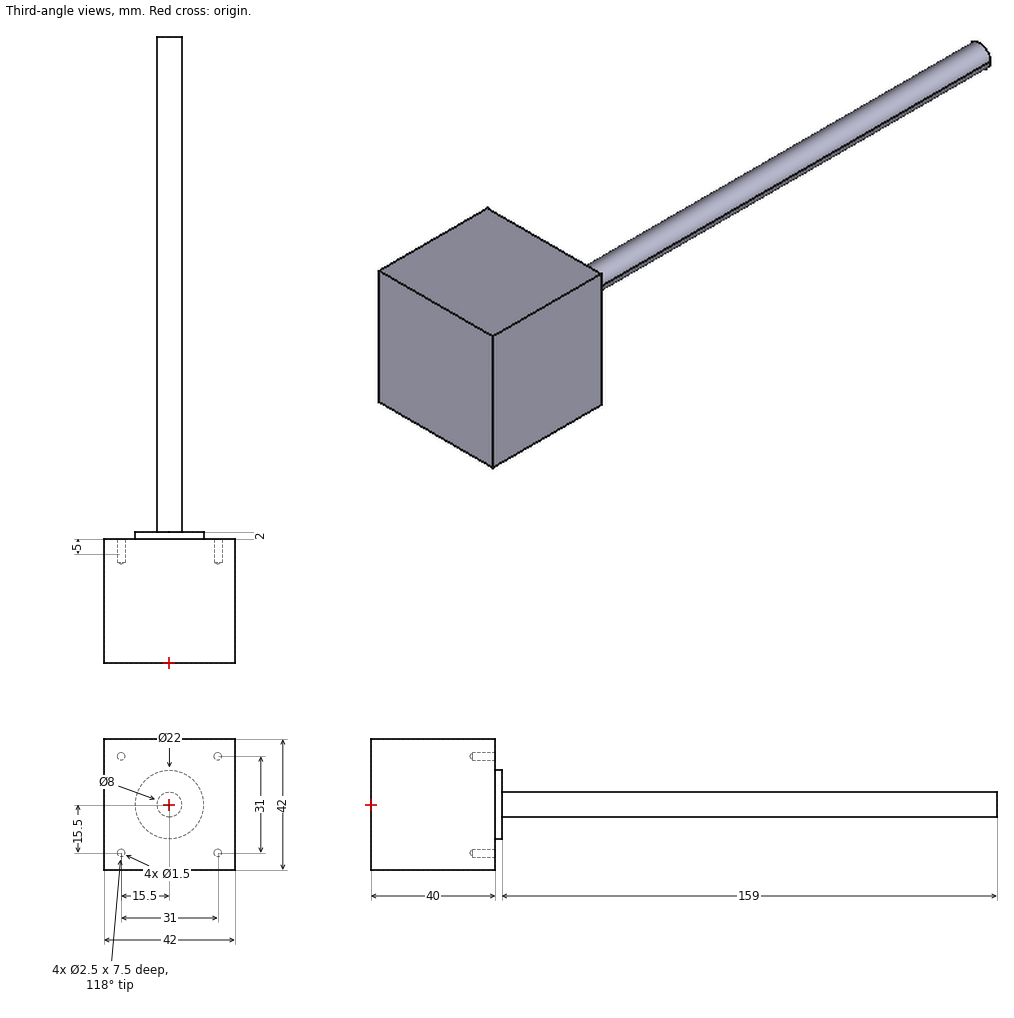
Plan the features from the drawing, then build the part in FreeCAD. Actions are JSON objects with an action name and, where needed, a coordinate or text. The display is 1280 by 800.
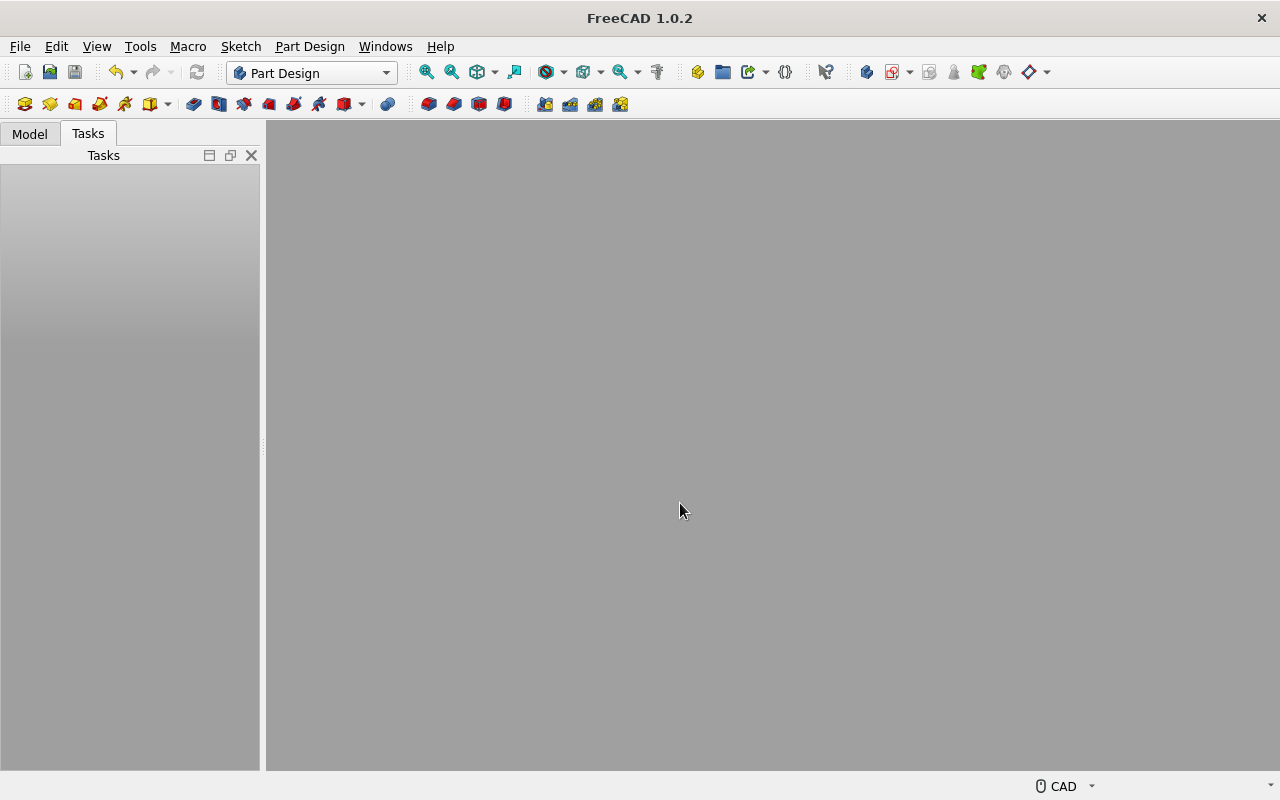
{"action": "left_click", "coordinate": [25, 72]}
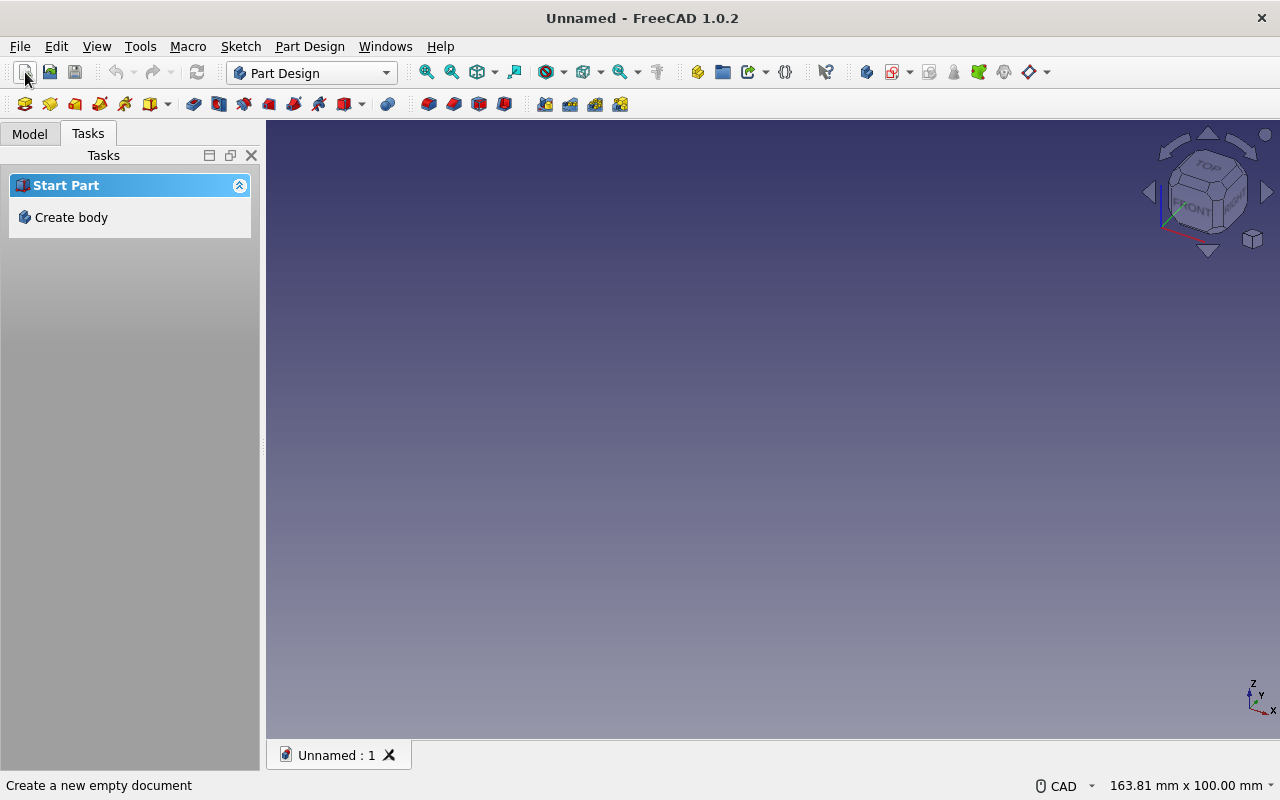
{"action": "left_click", "coordinate": [892, 72]}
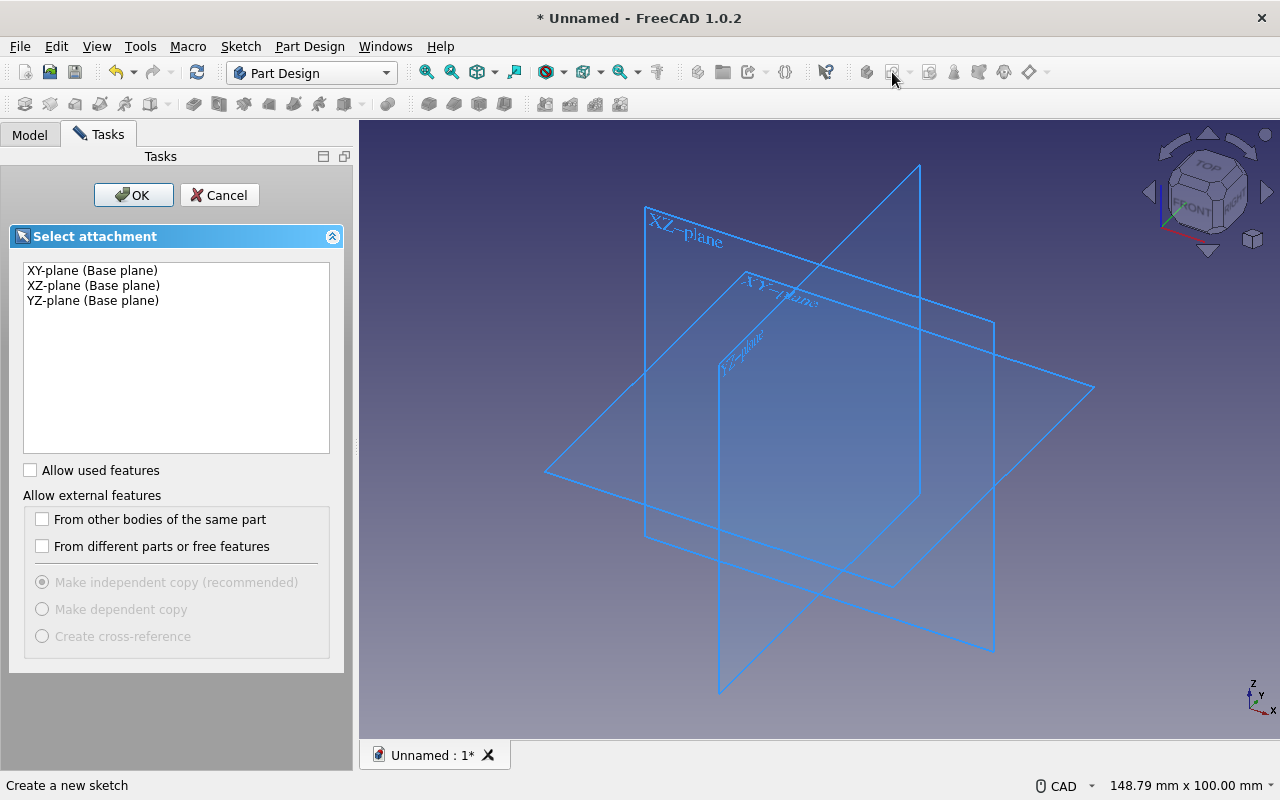
{"action": "left_click", "coordinate": [84, 286]}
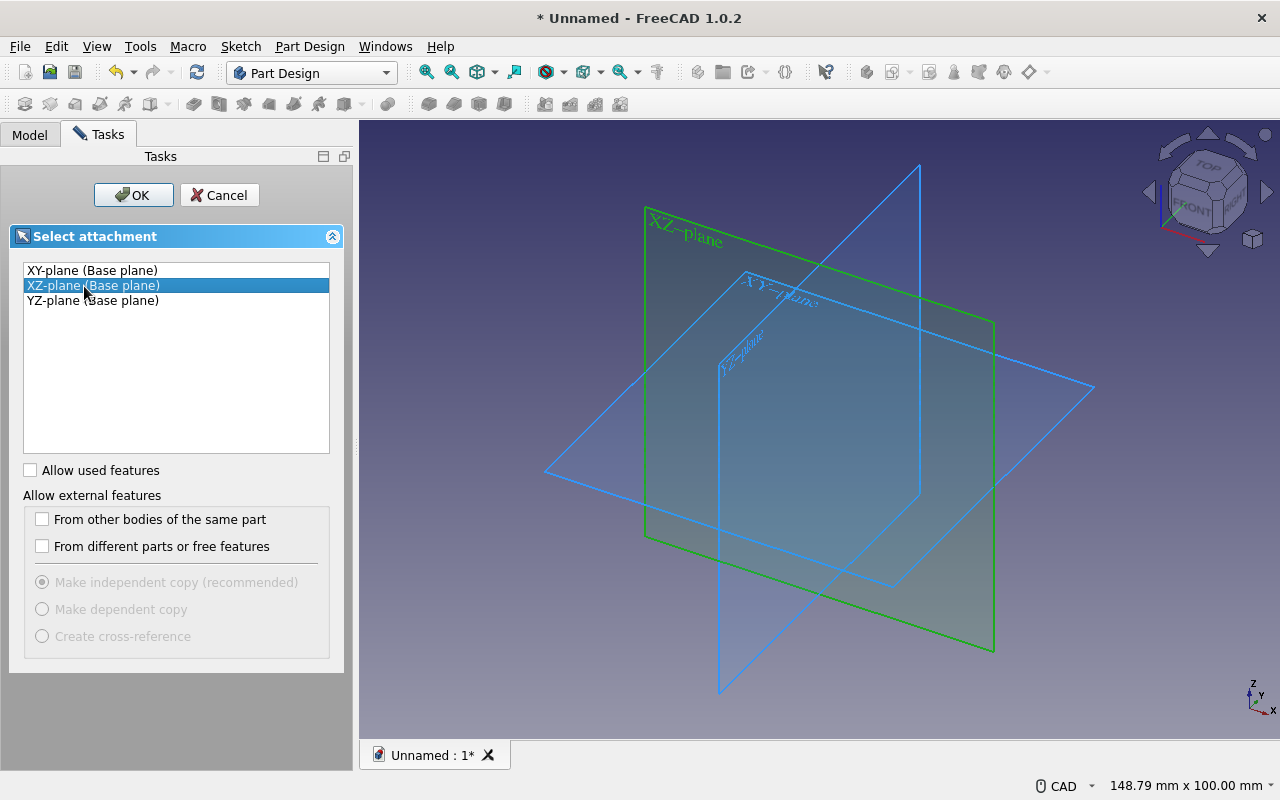
{"action": "left_click", "coordinate": [134, 195]}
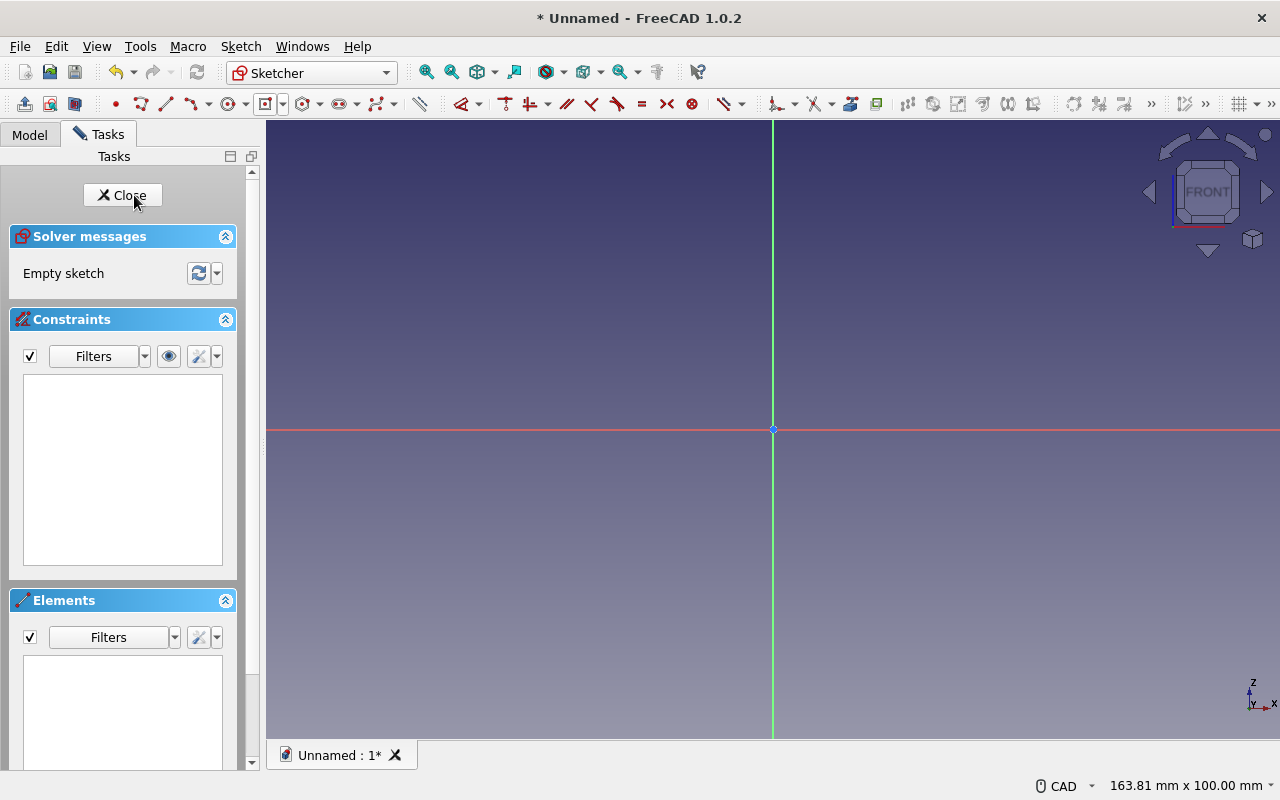
{"action": "scroll", "coordinate": [912, 429], "scroll_direction": "up", "scroll_amount": 2}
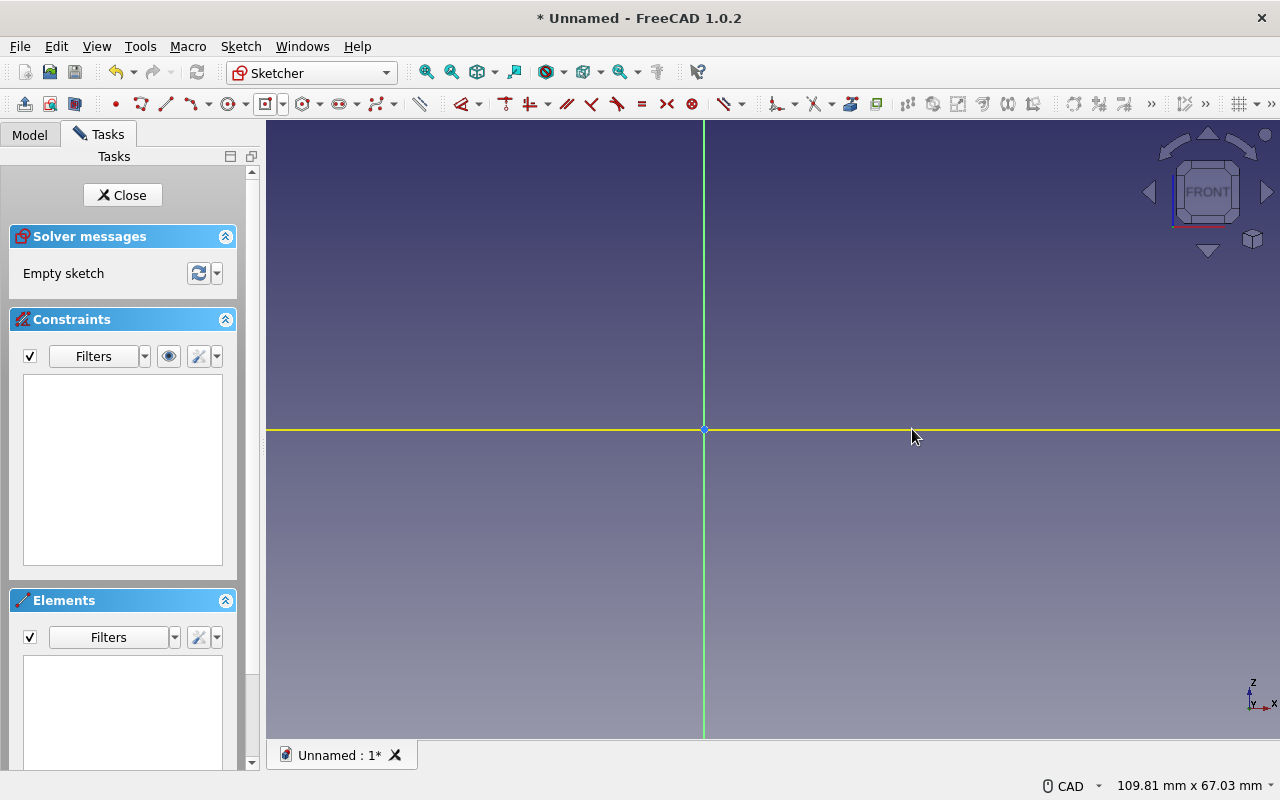
{"action": "left_click", "coordinate": [264, 104]}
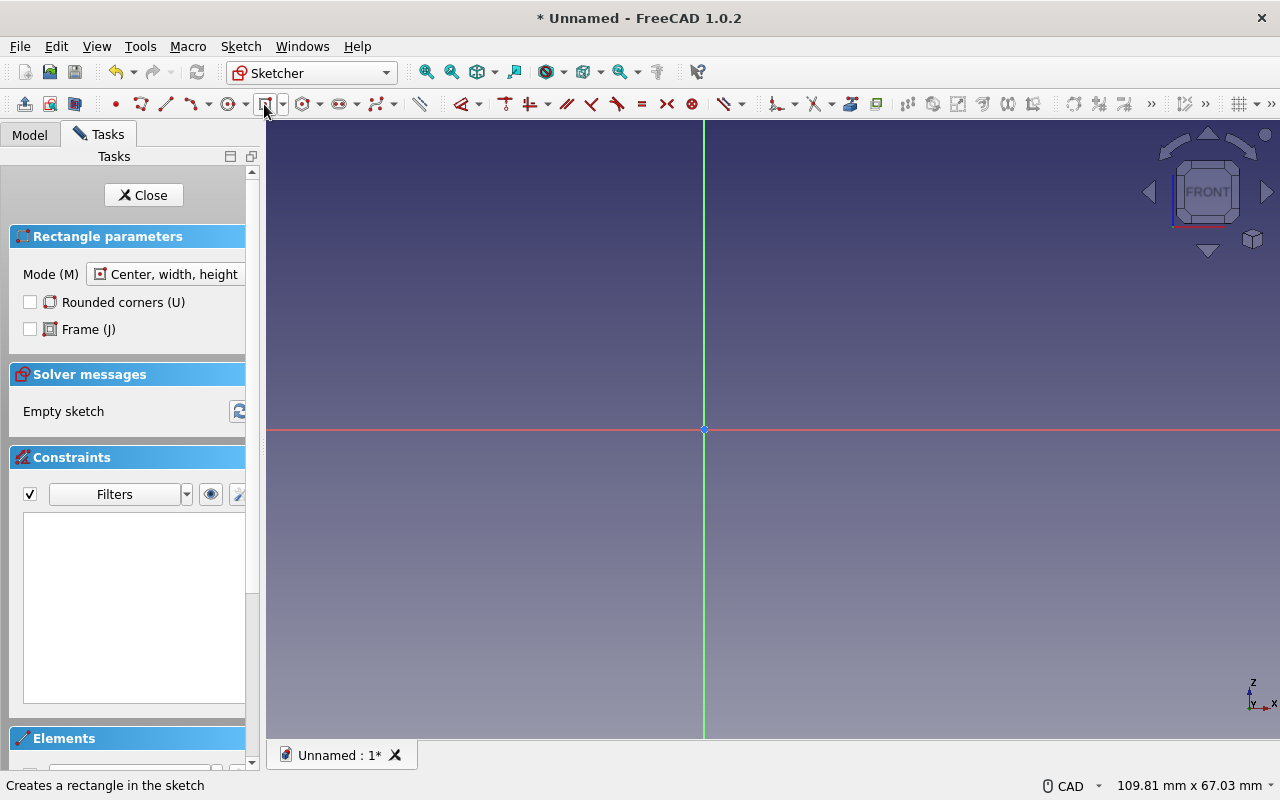
{"action": "left_click", "coordinate": [704, 430]}
{"action": "left_click", "coordinate": [898, 236]}
{"action": "key", "text": "Escape"}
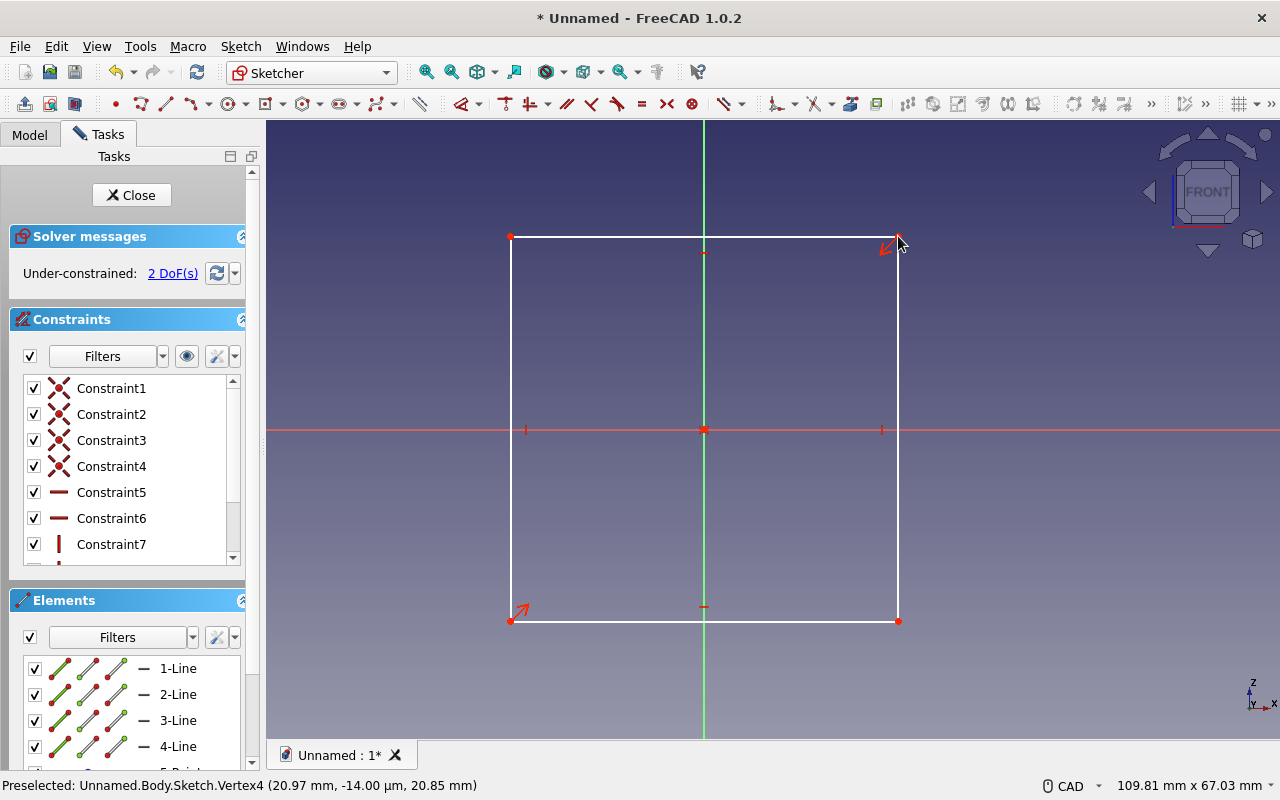
{"action": "left_click", "coordinate": [627, 622]}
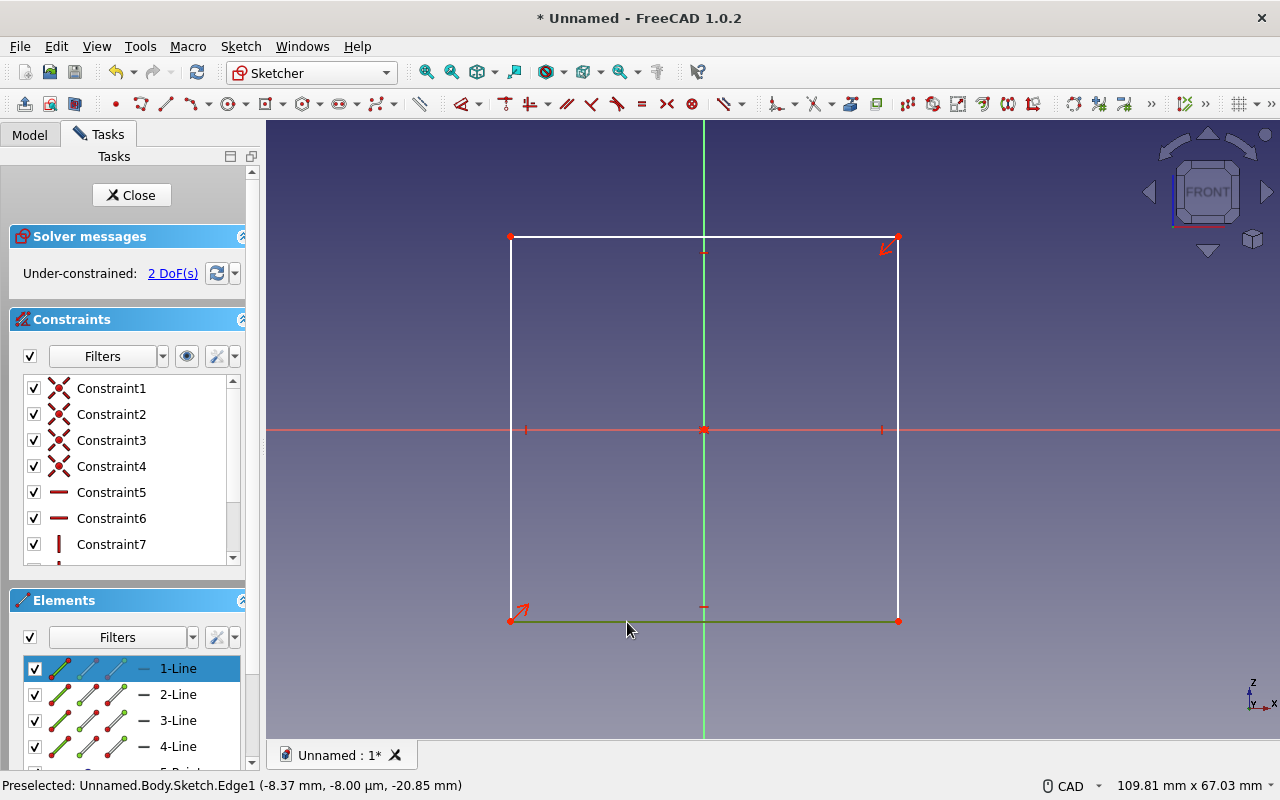
{"action": "left_click", "coordinate": [478, 104]}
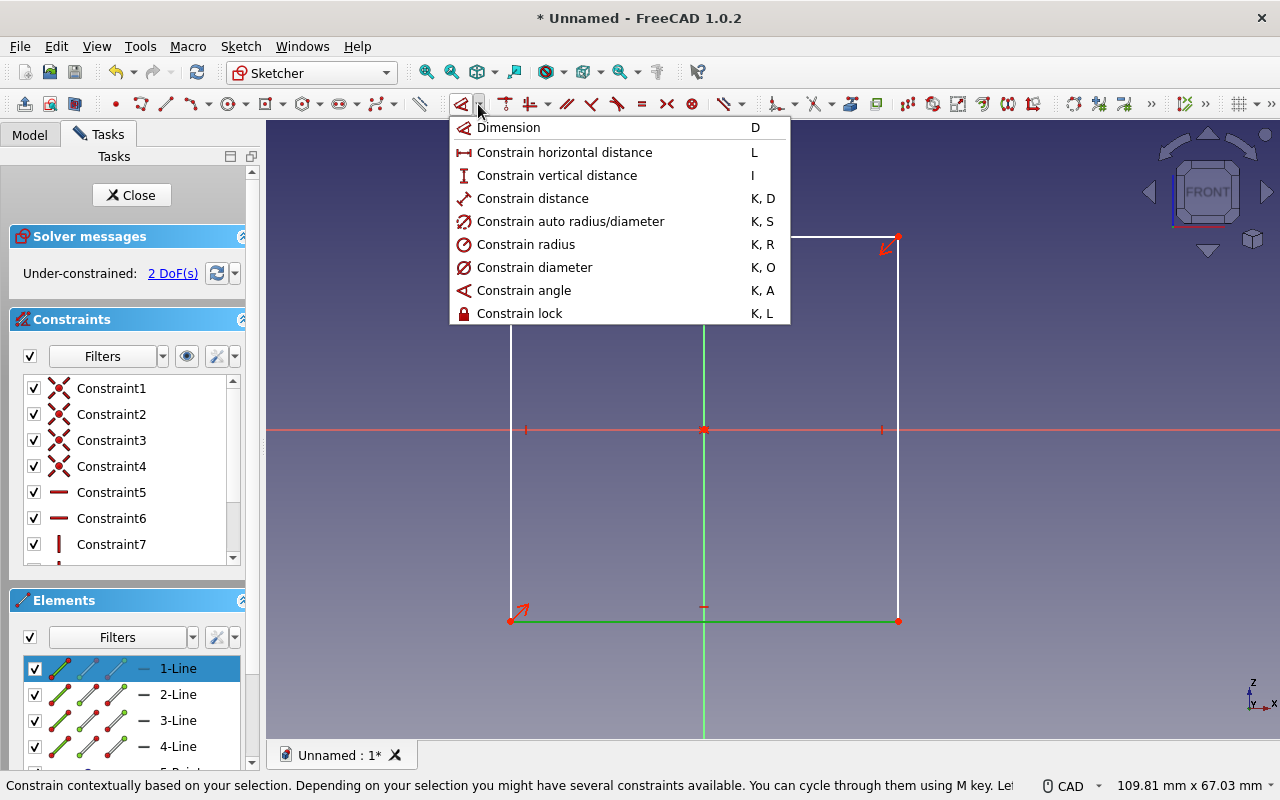
{"action": "left_click", "coordinate": [620, 152]}